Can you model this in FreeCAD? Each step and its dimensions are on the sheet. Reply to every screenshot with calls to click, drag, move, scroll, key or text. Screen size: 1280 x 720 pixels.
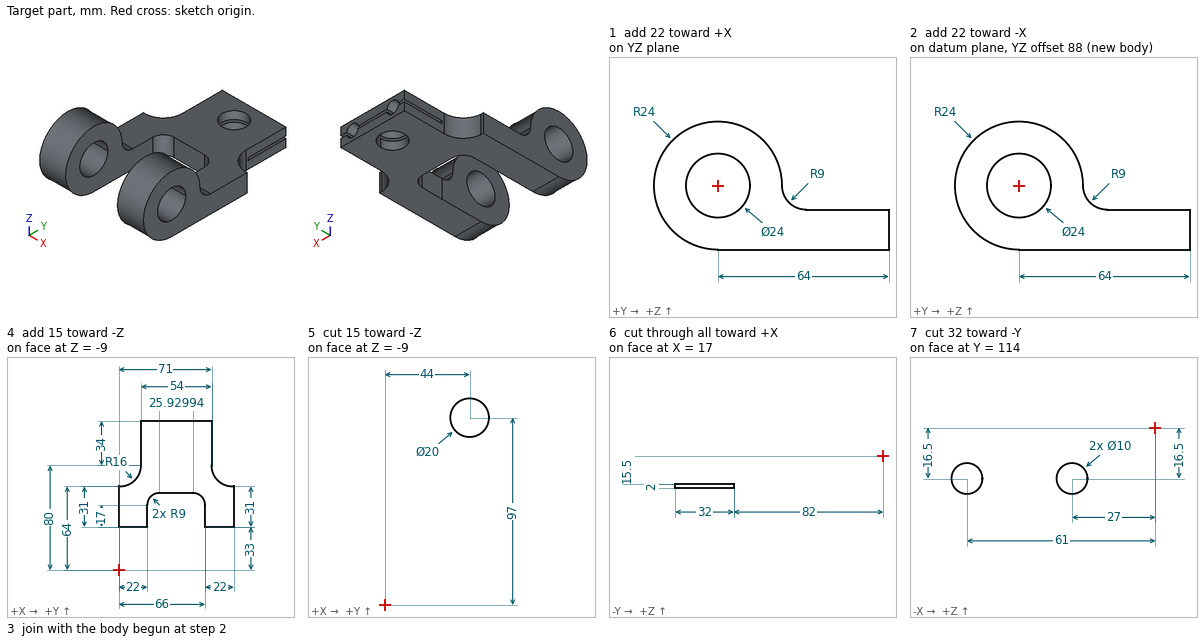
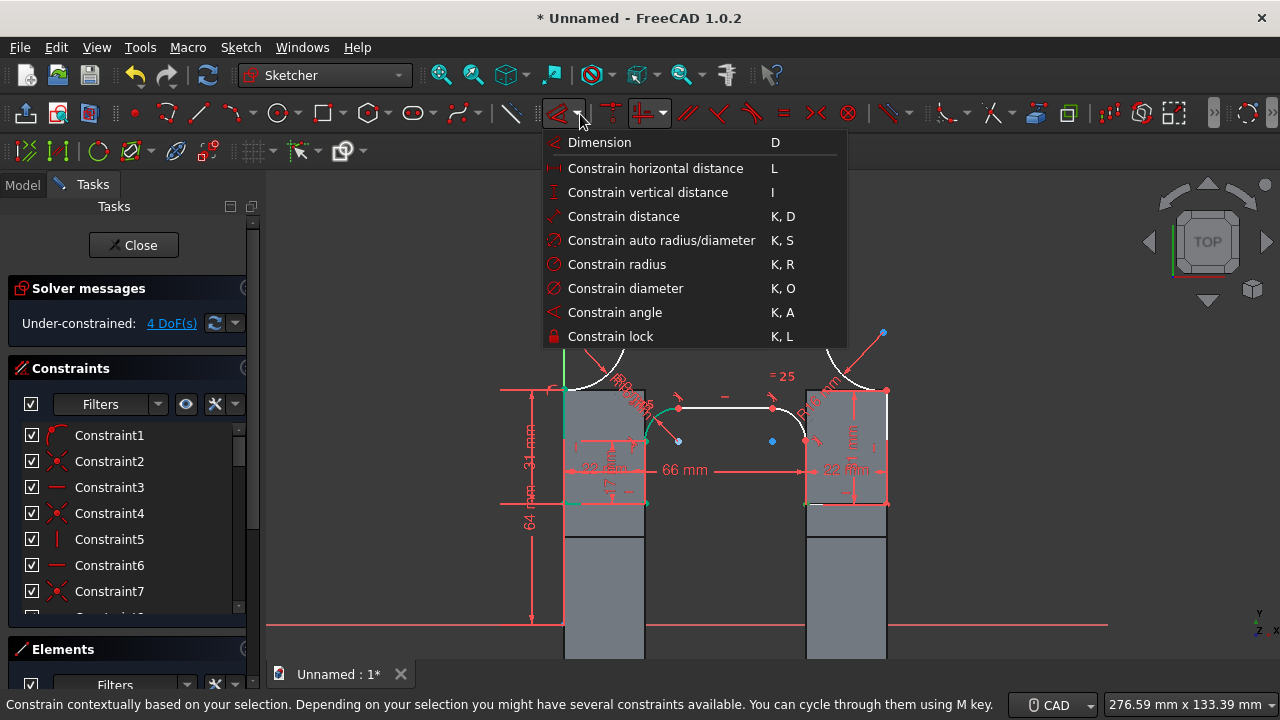
click(695, 192)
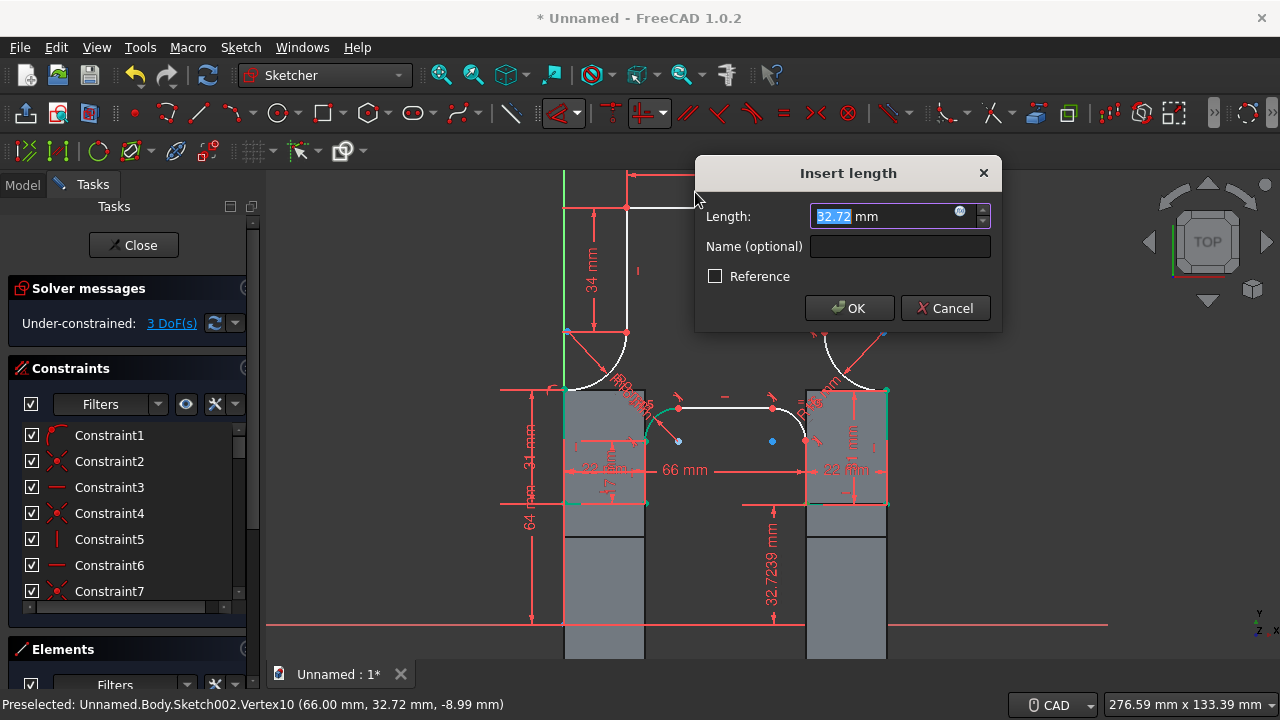
text(33)
key(Return)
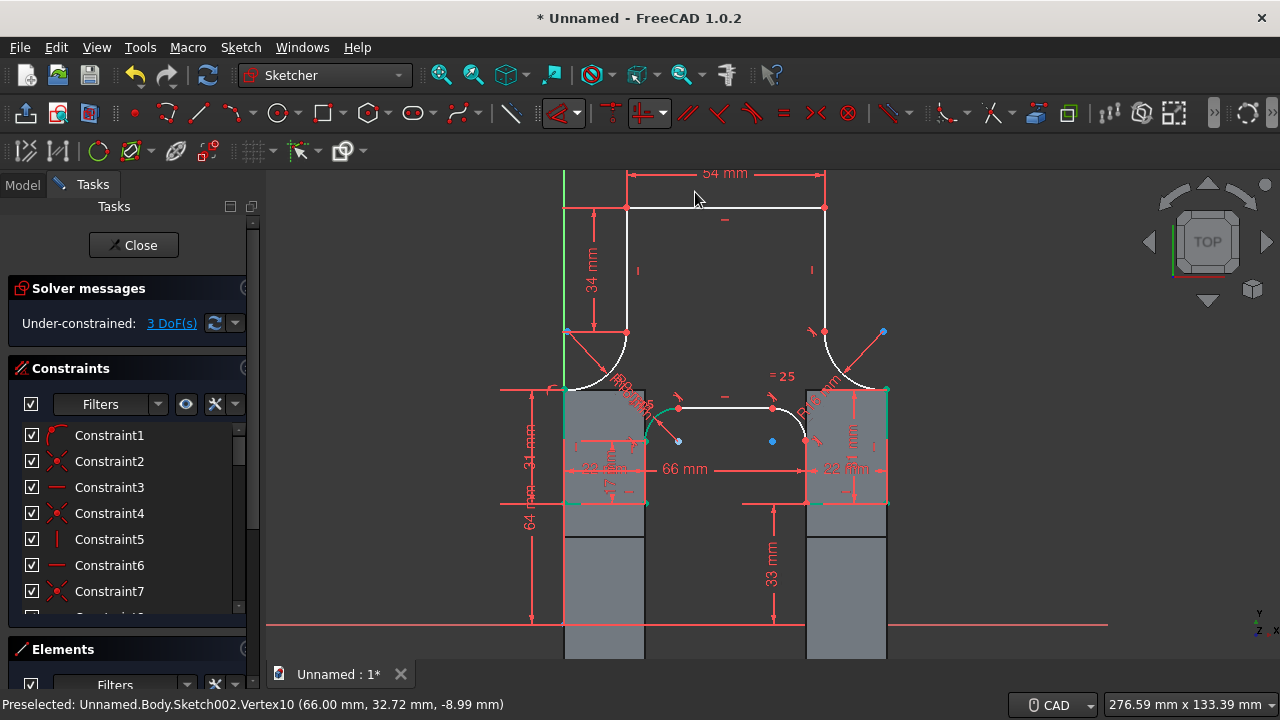
click(825, 331)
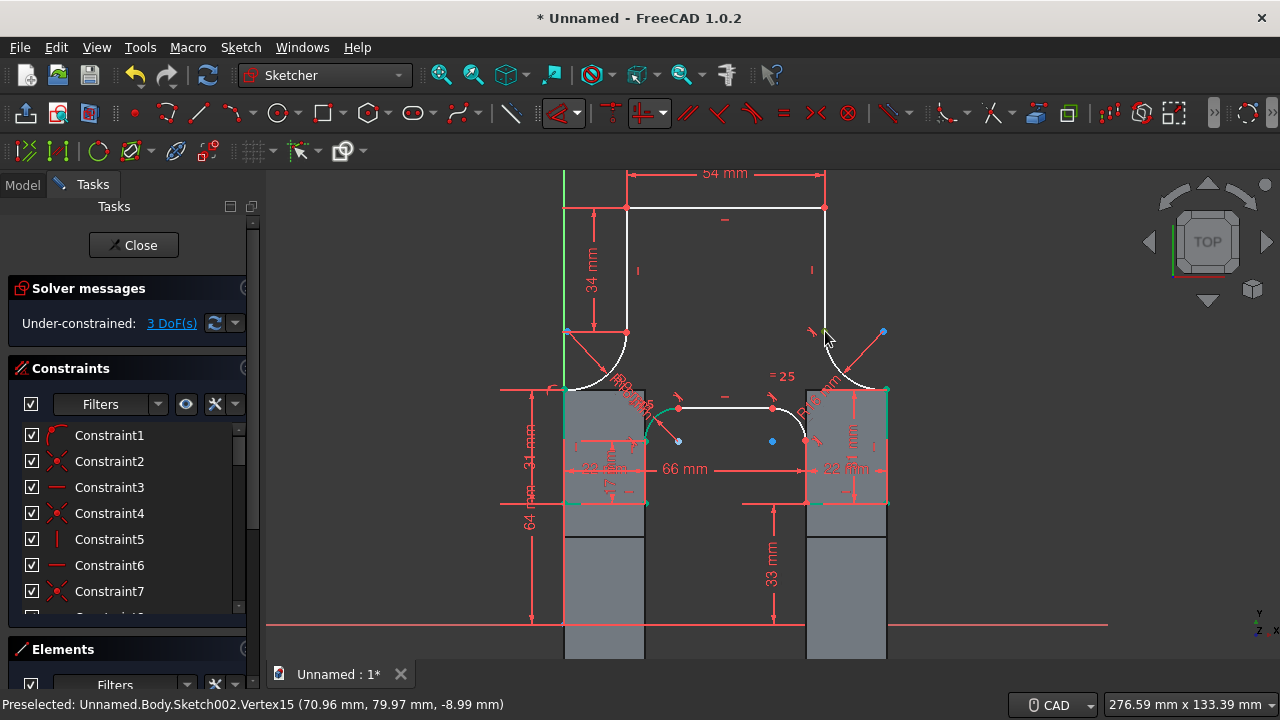
key(l)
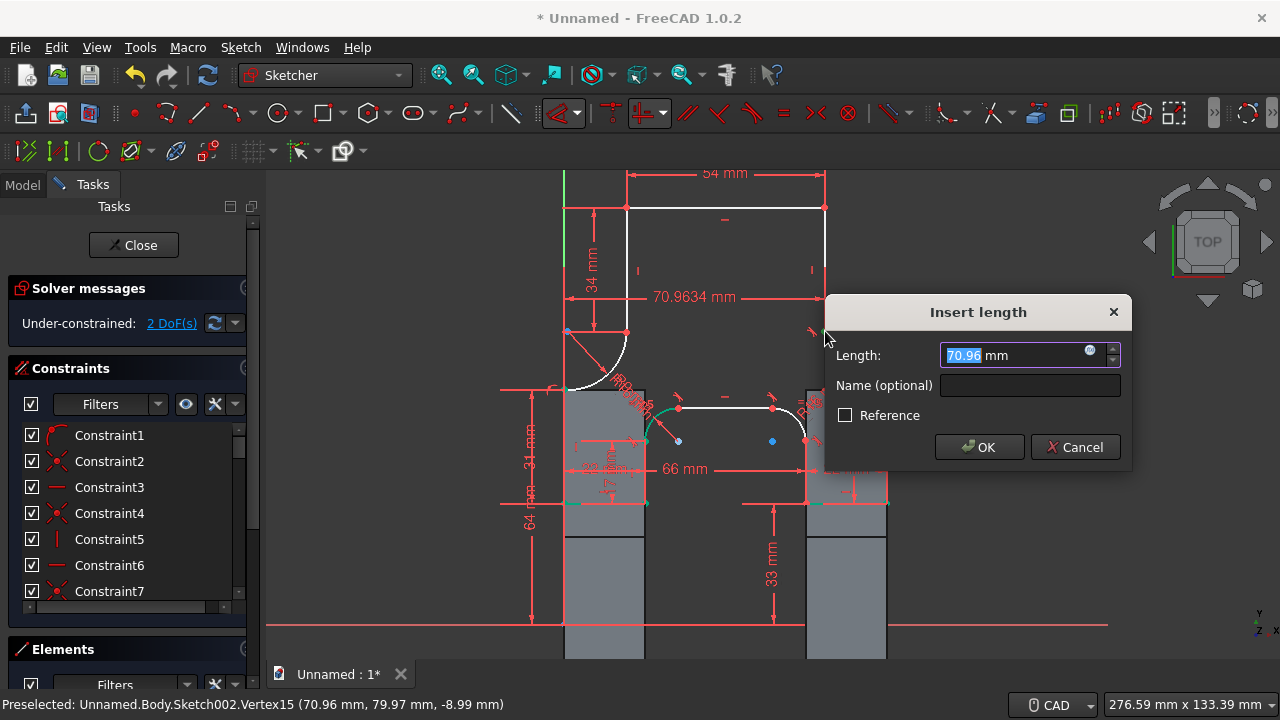
text(71)
key(Return)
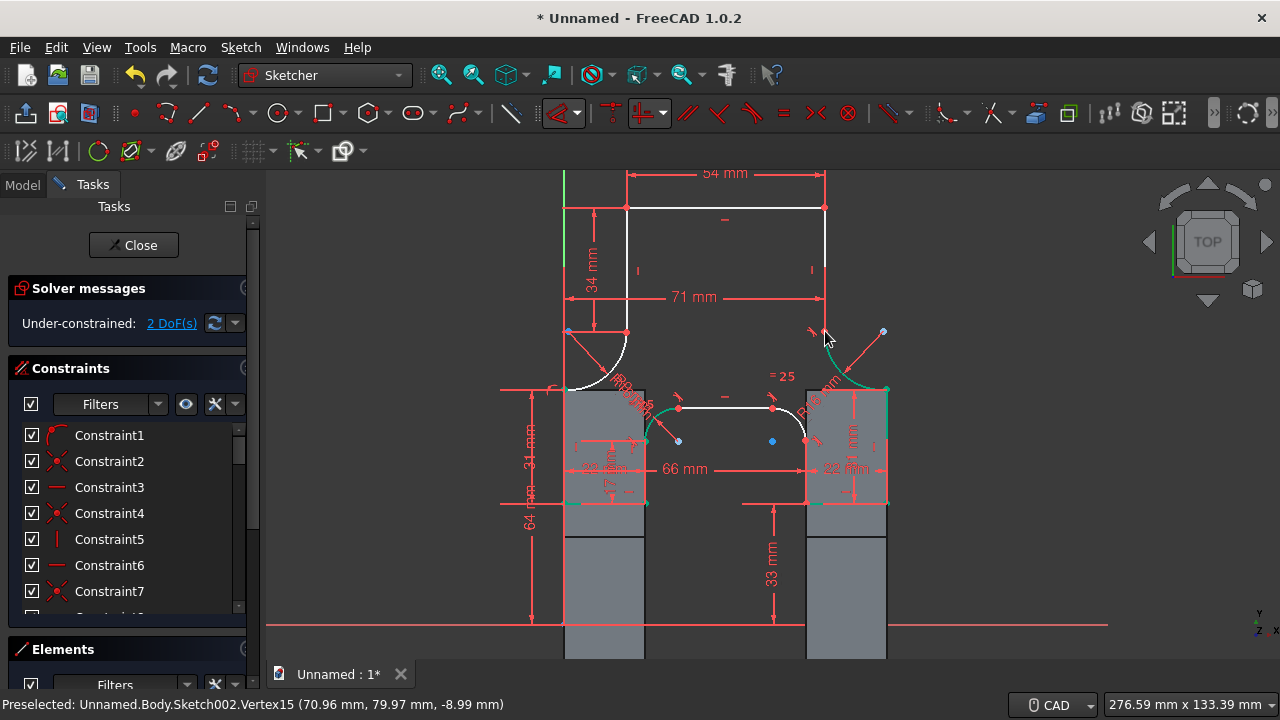
click(627, 332)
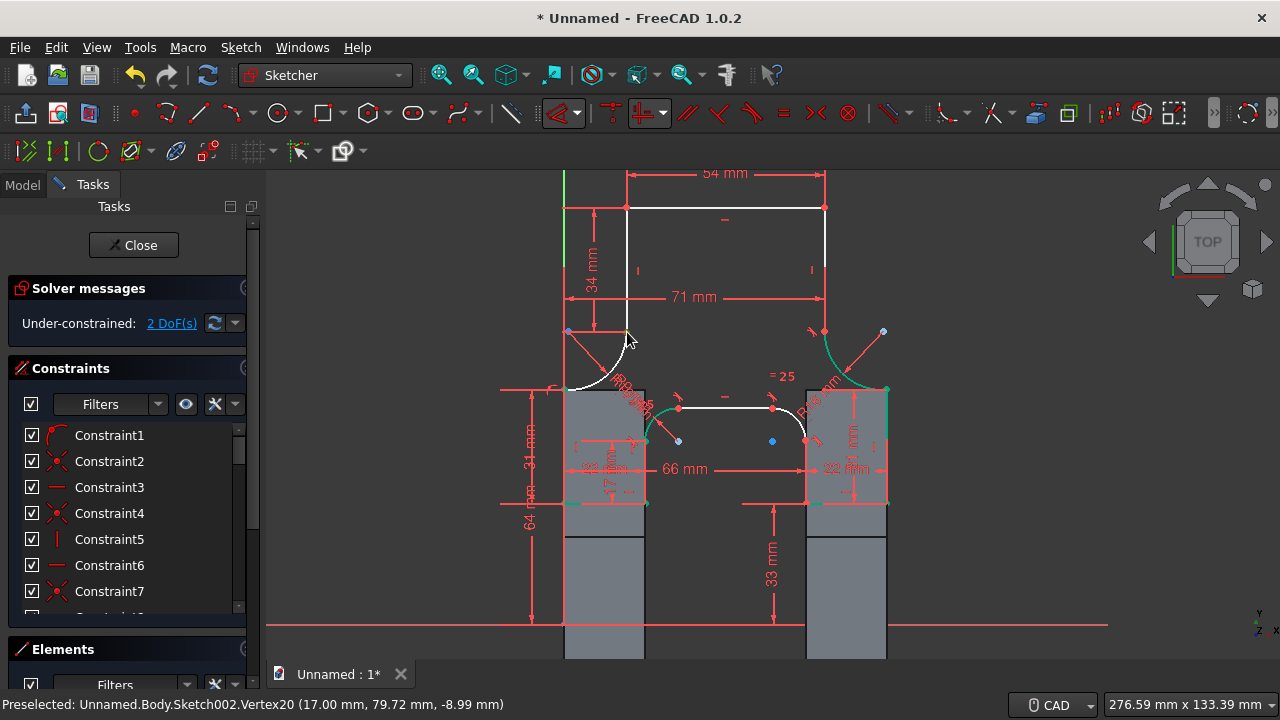
click(580, 114)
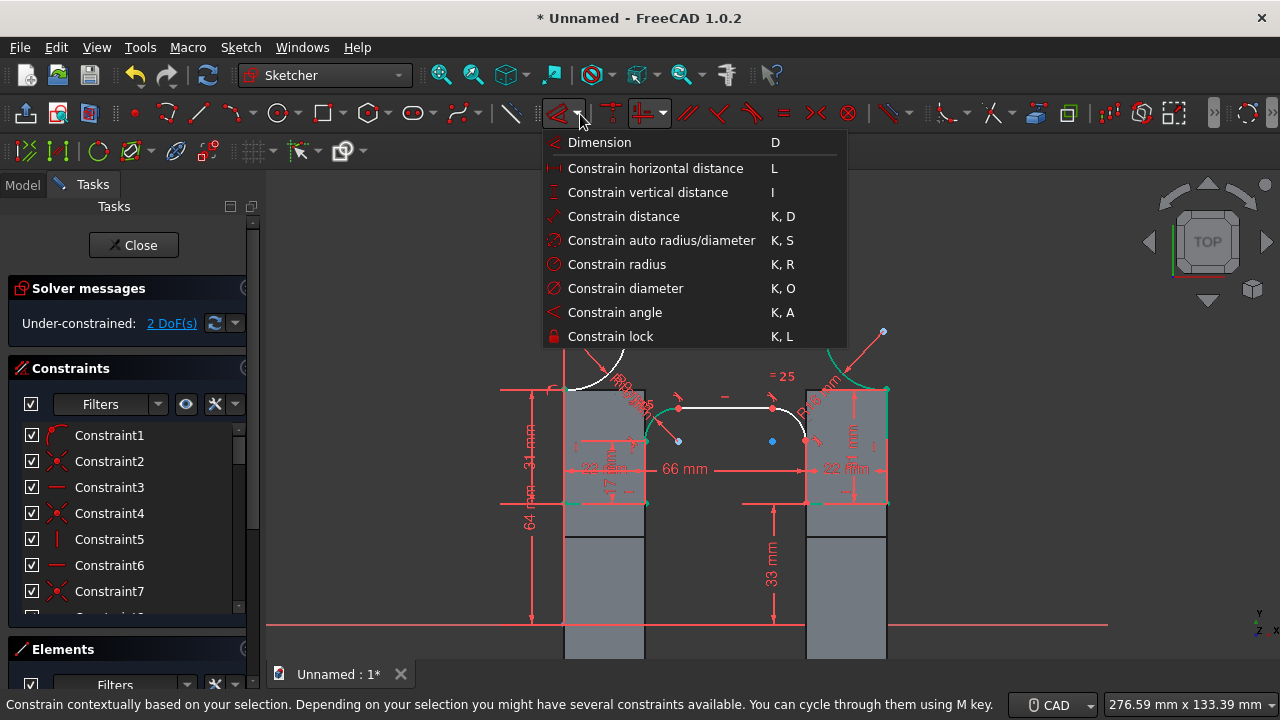
click(695, 192)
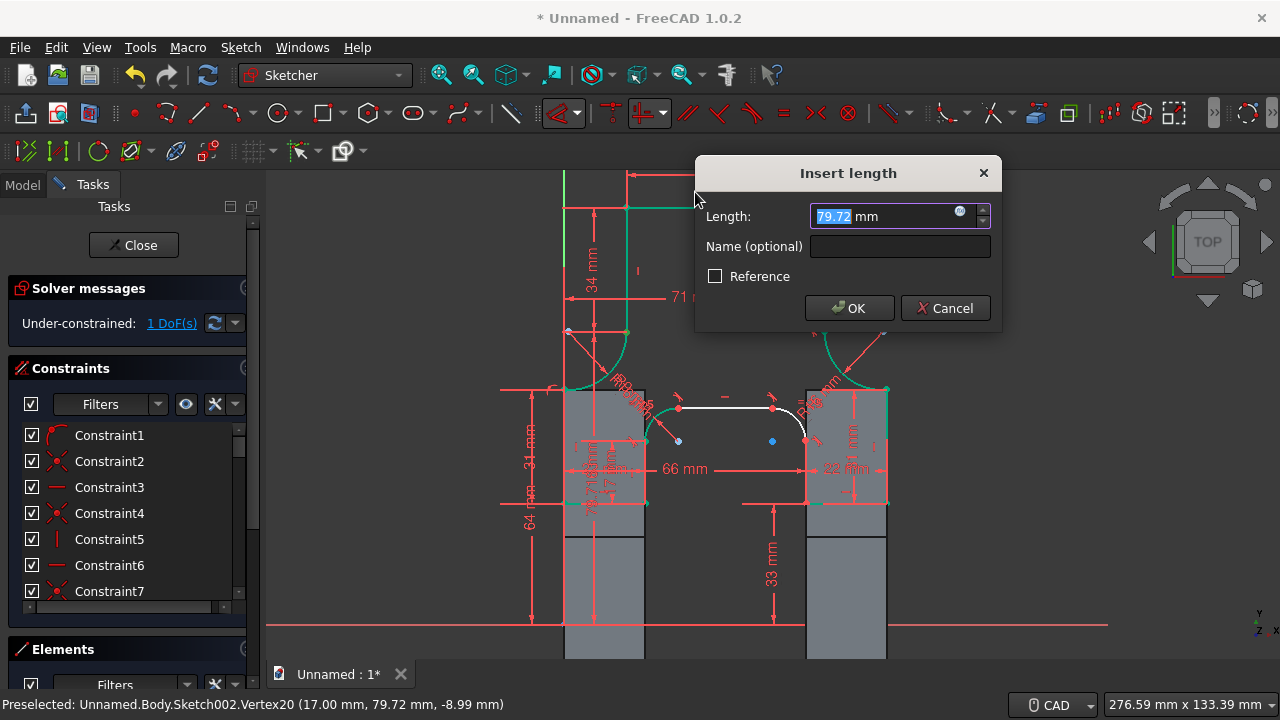
text(80)
key(Return)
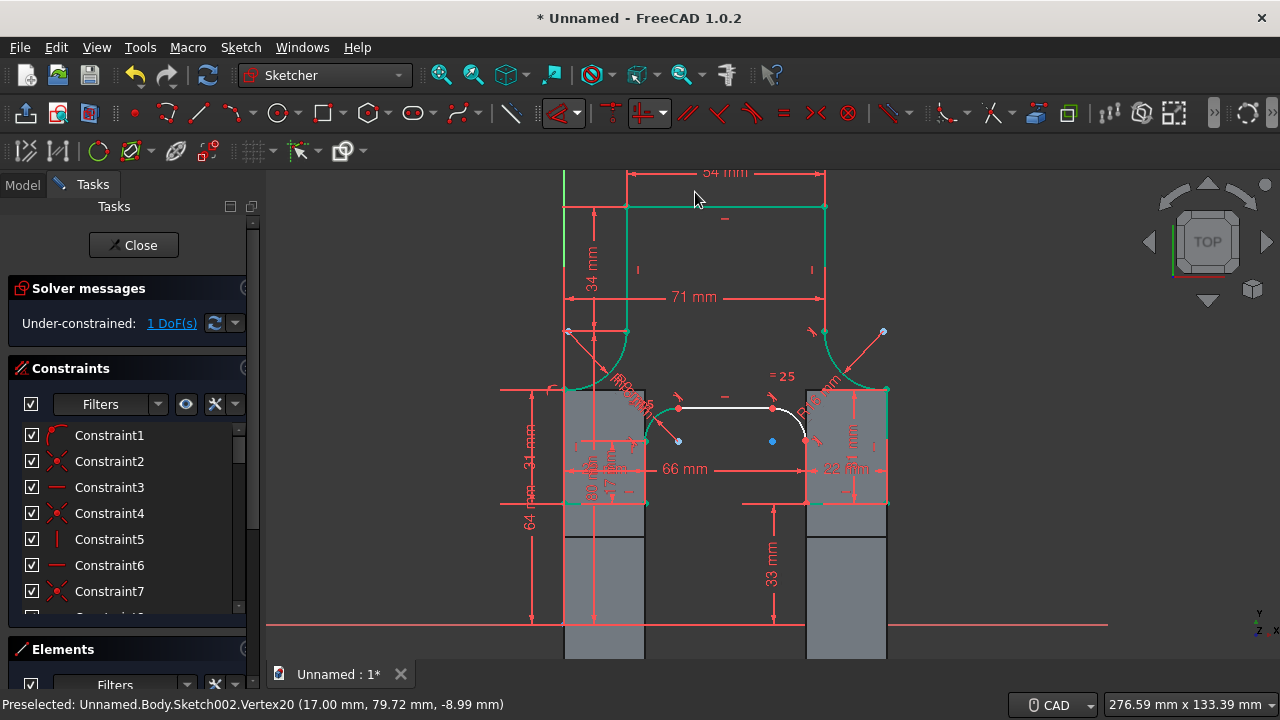
click(706, 408)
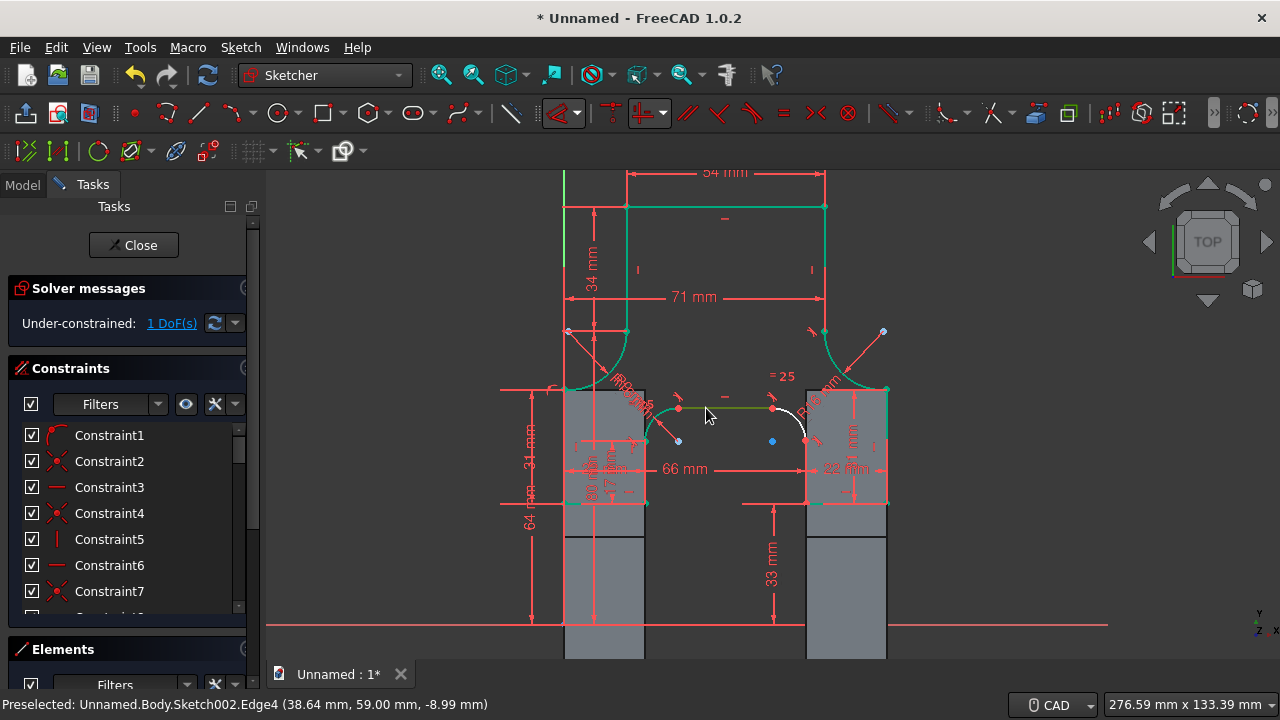
click(580, 114)